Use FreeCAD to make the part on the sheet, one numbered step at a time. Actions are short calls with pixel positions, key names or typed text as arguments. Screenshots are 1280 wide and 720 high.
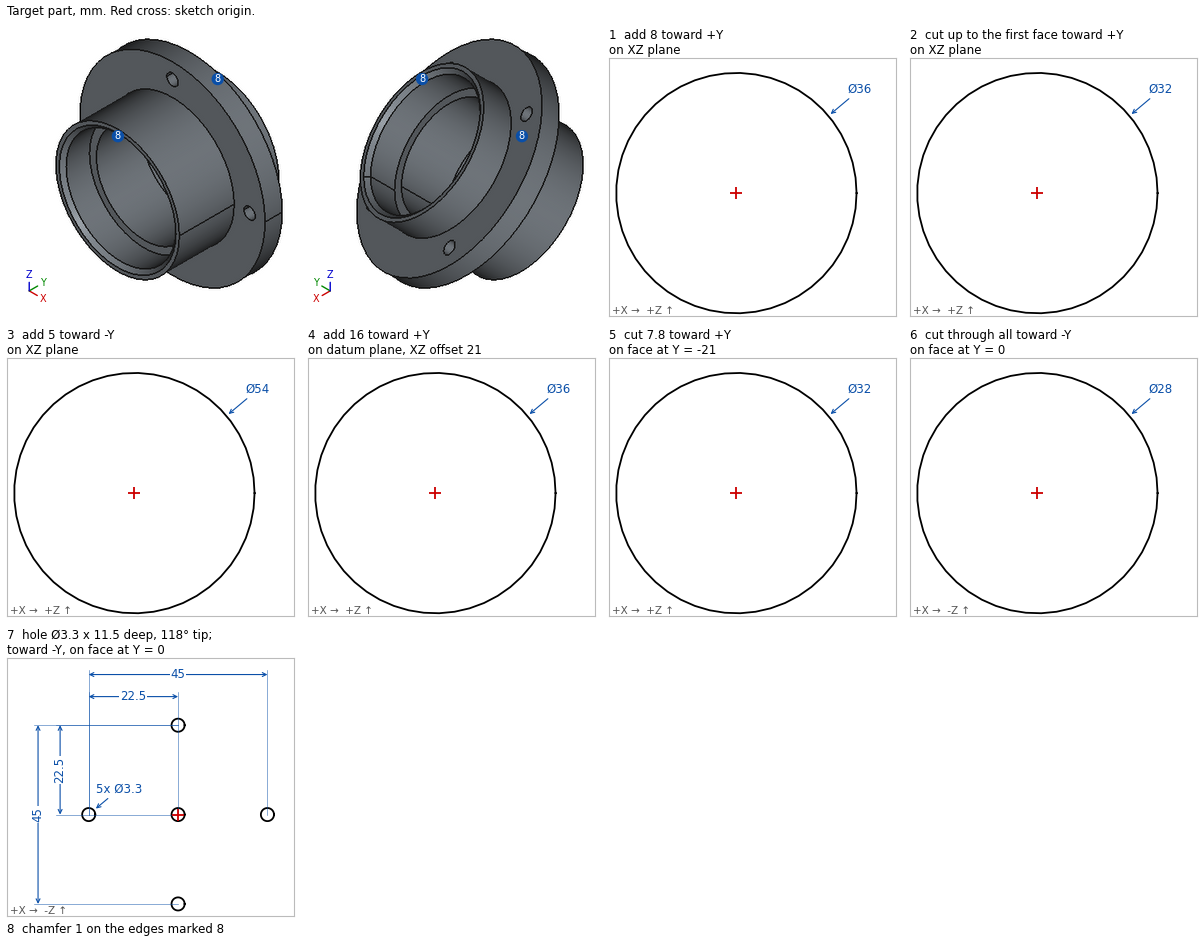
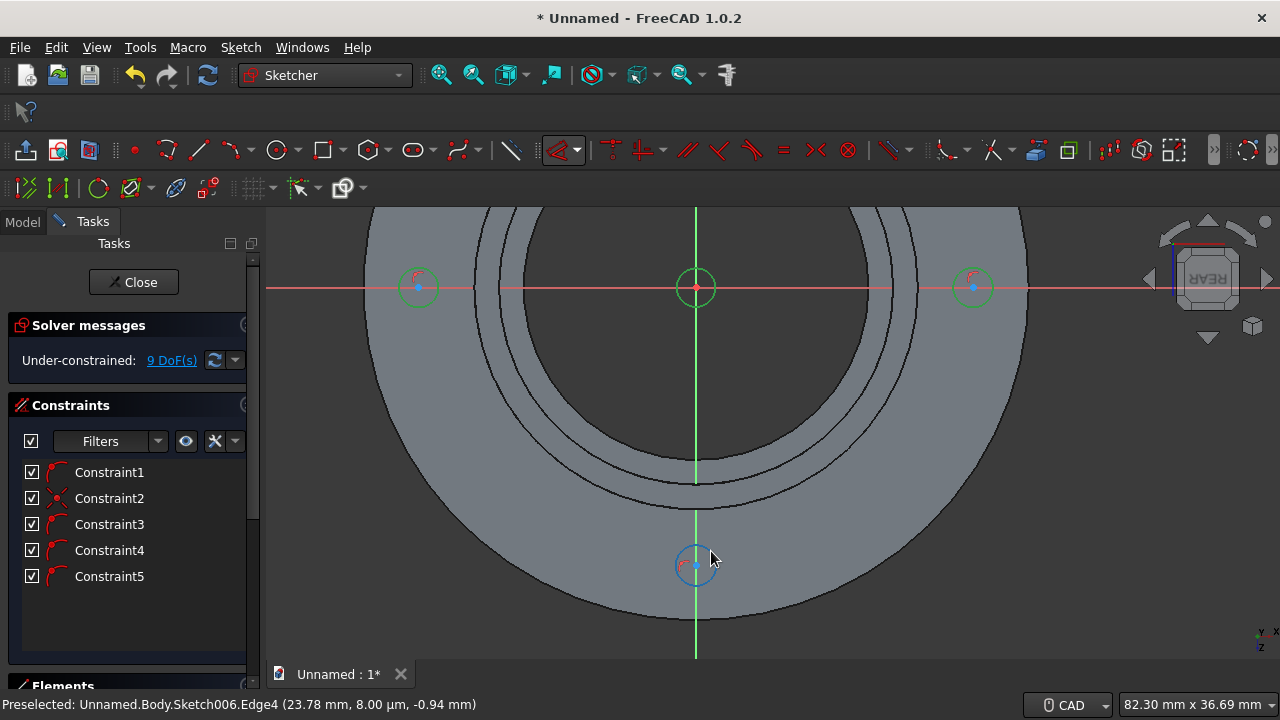
click(710, 551)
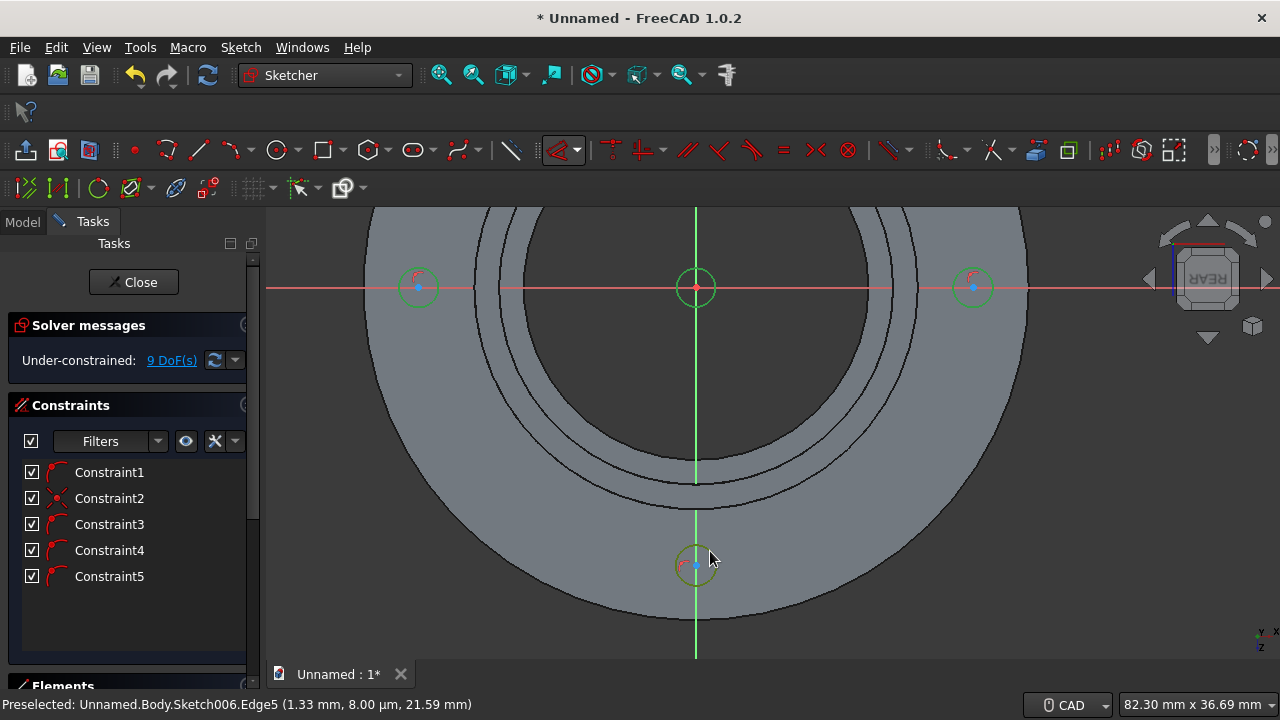
click(784, 150)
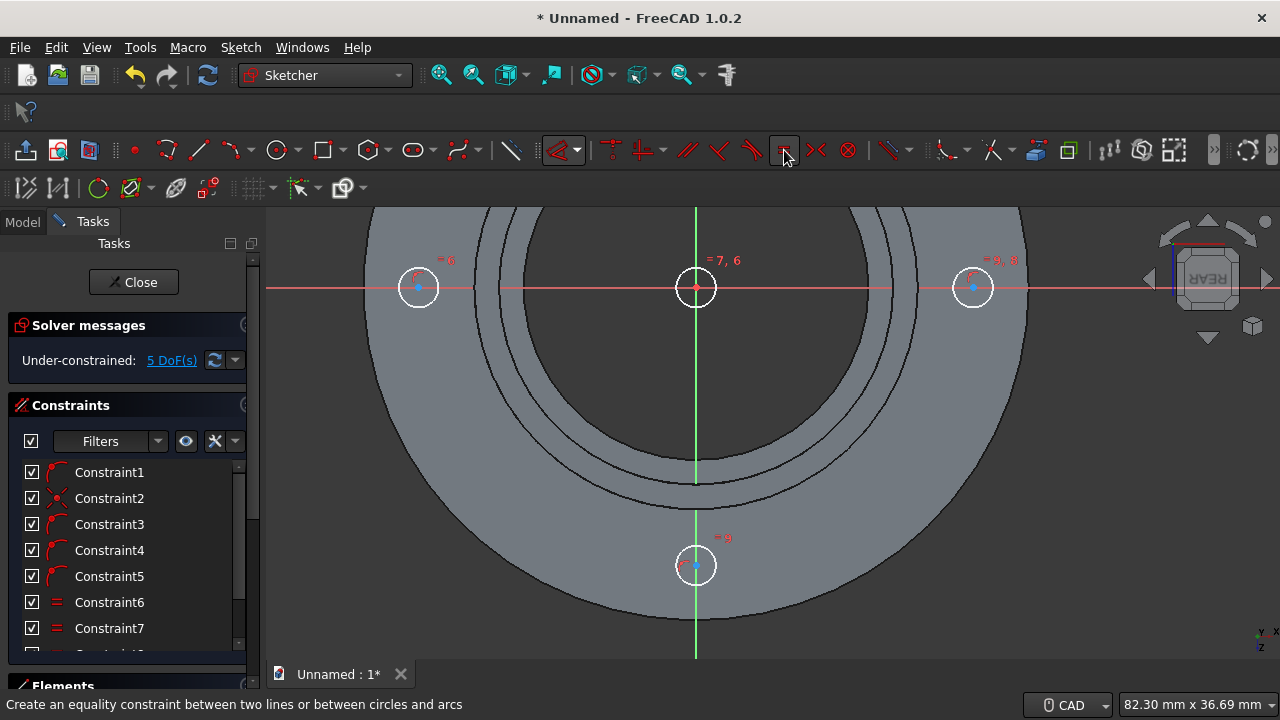
click(433, 274)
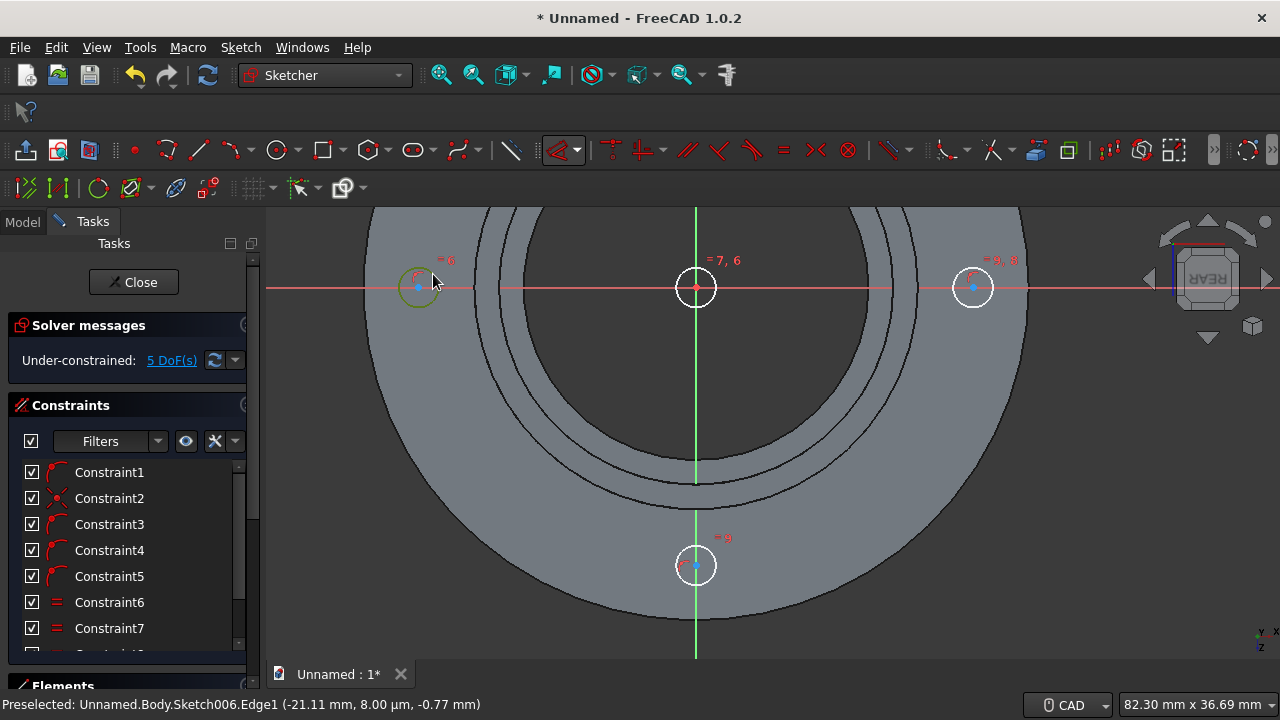
click(580, 150)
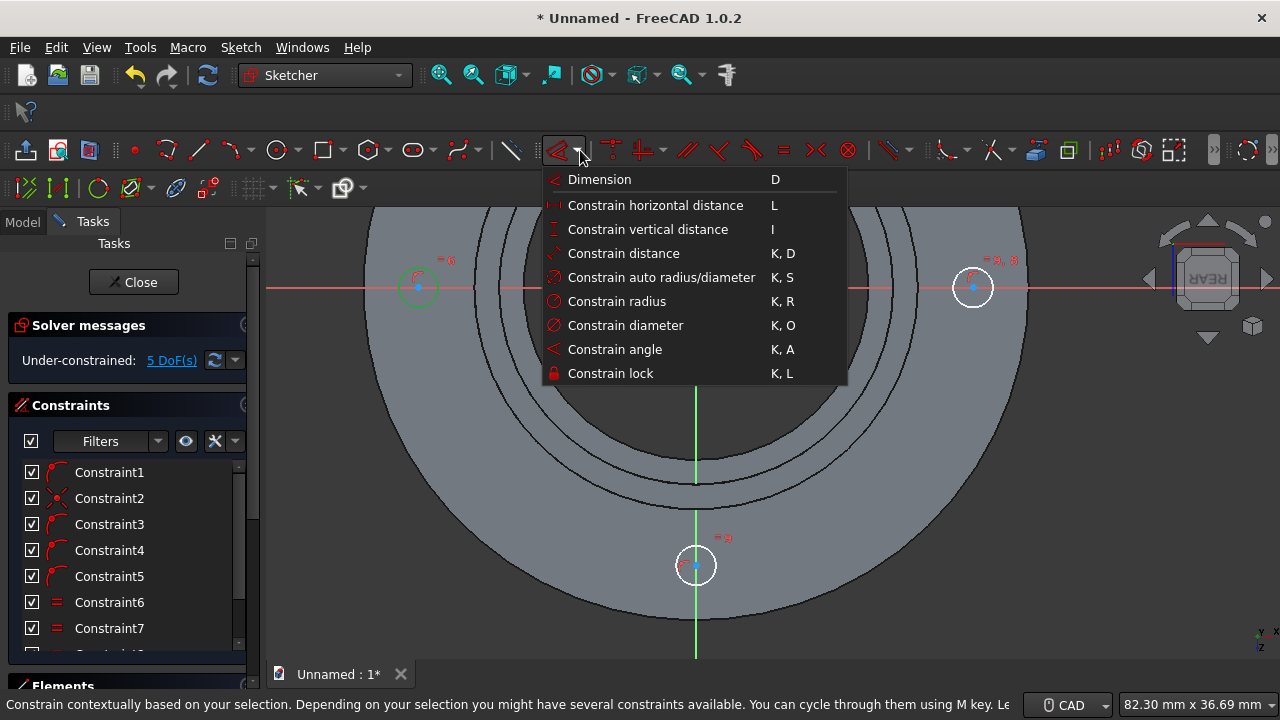
click(695, 325)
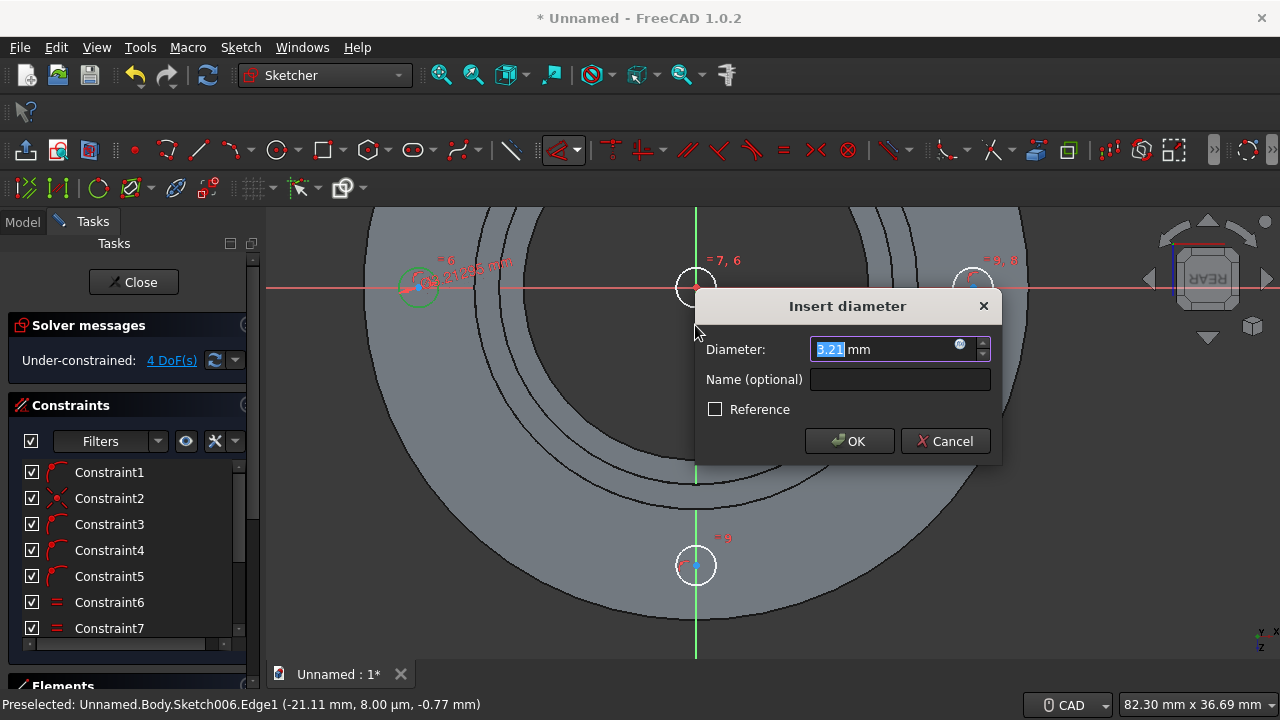
text(3.3)
key(Return)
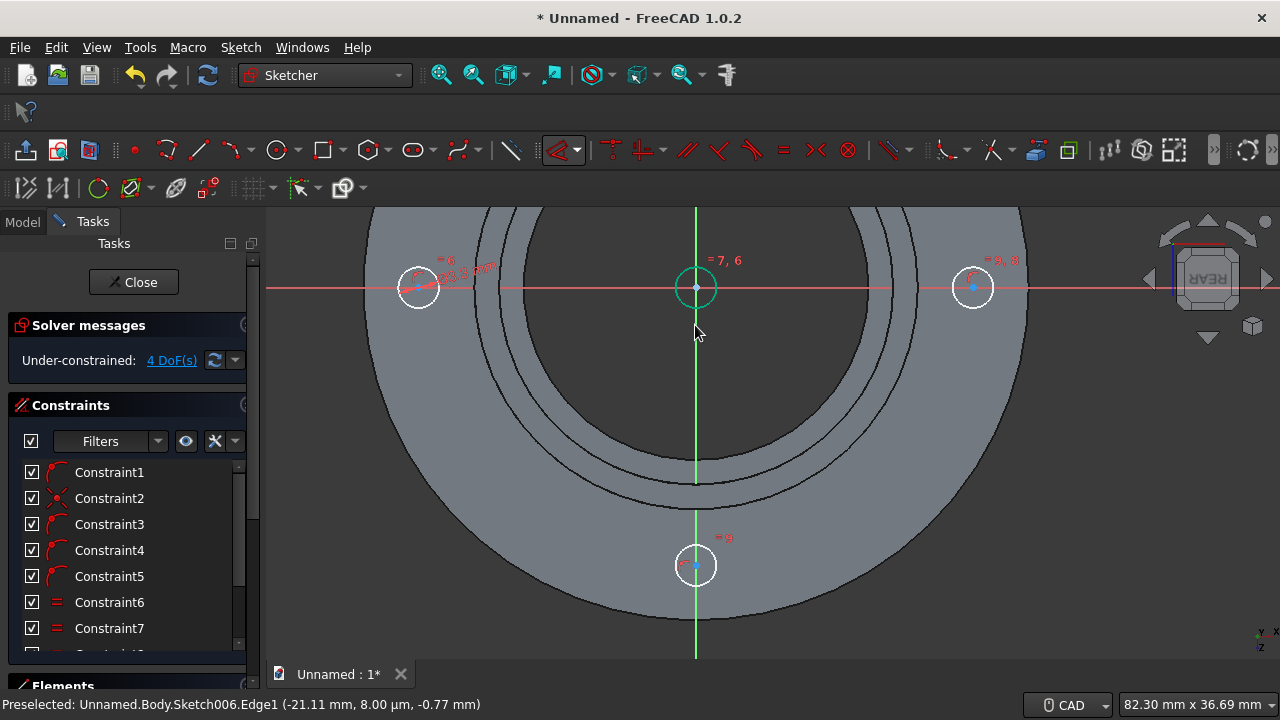
click(419, 288)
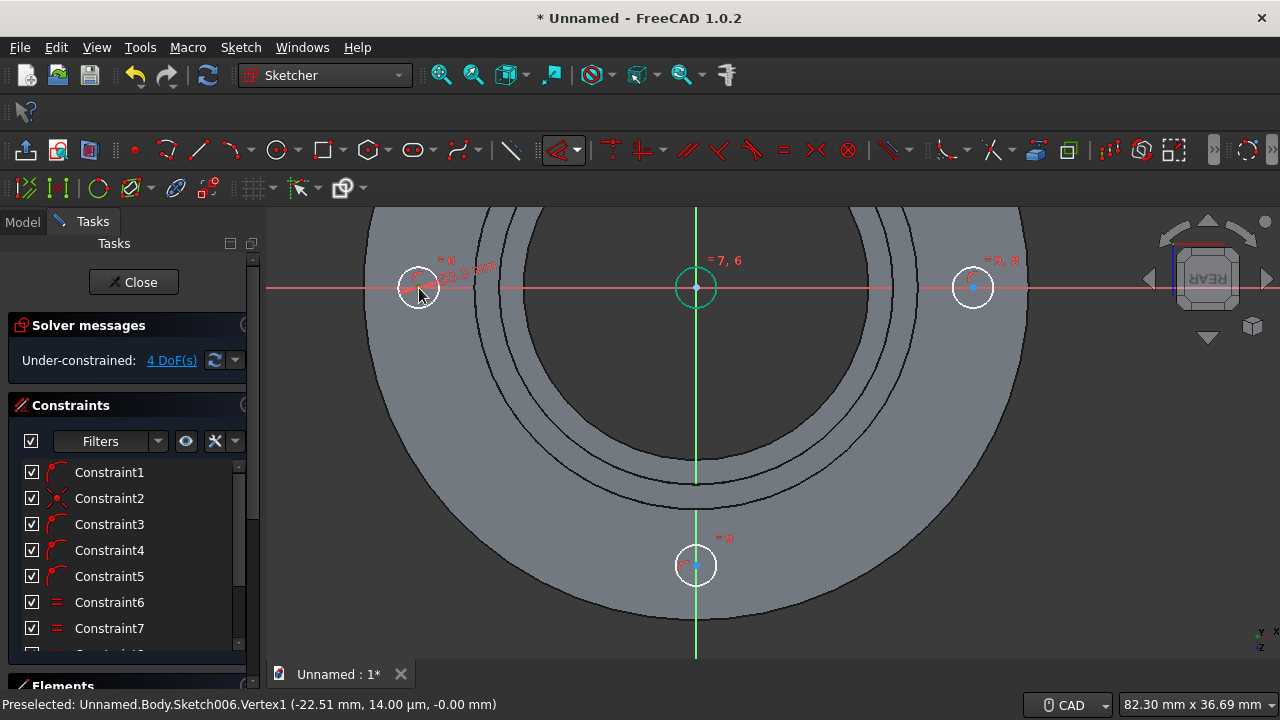
click(973, 288)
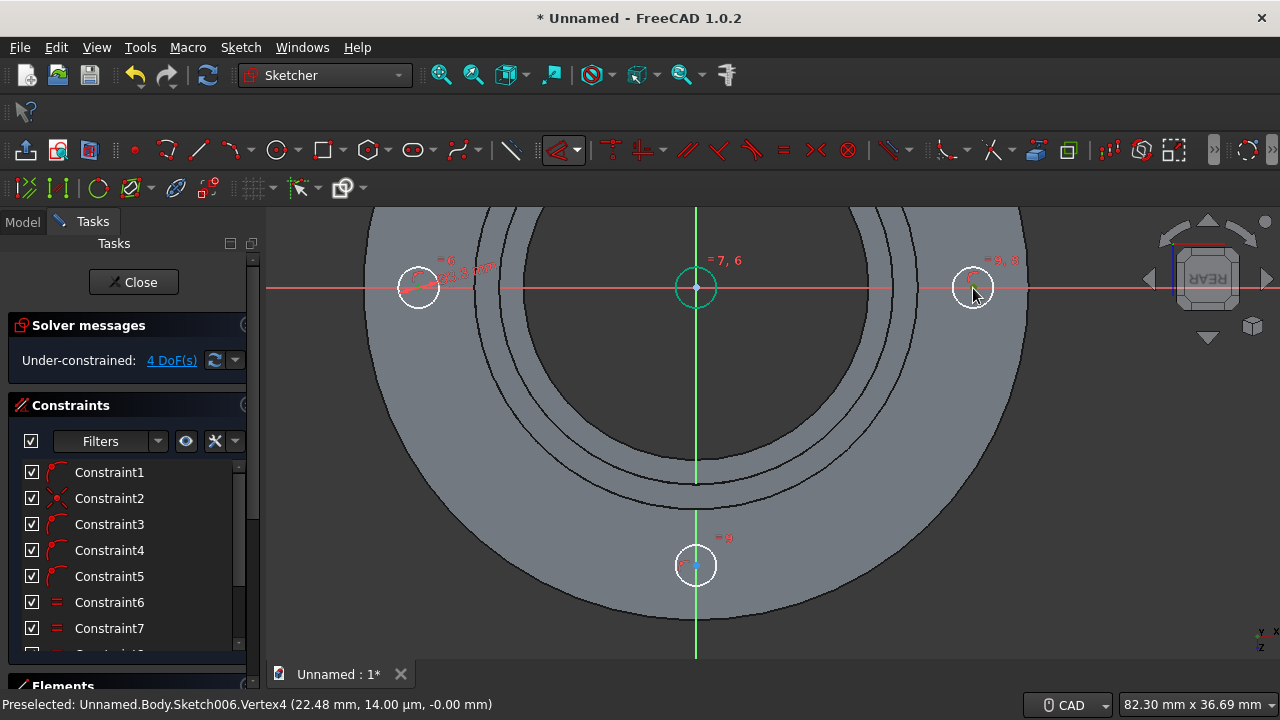
key(l)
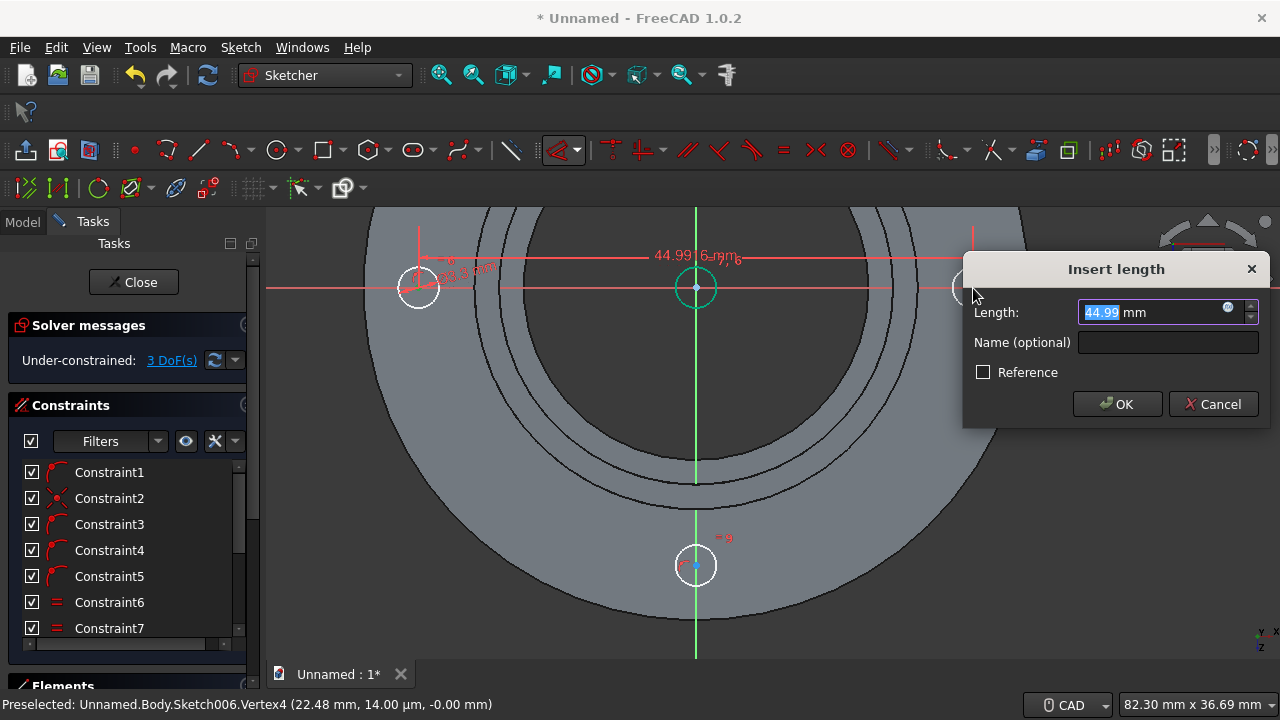
text(45)
key(Return)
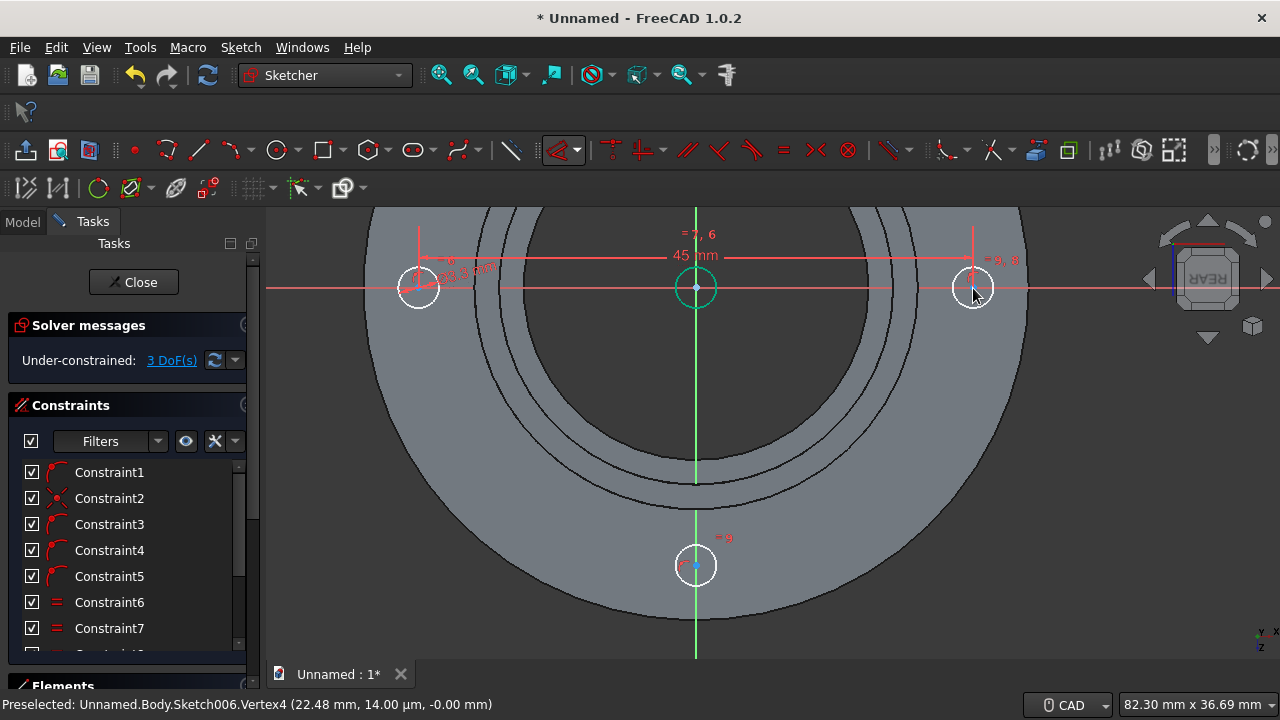
scroll(711, 552, down, 4)